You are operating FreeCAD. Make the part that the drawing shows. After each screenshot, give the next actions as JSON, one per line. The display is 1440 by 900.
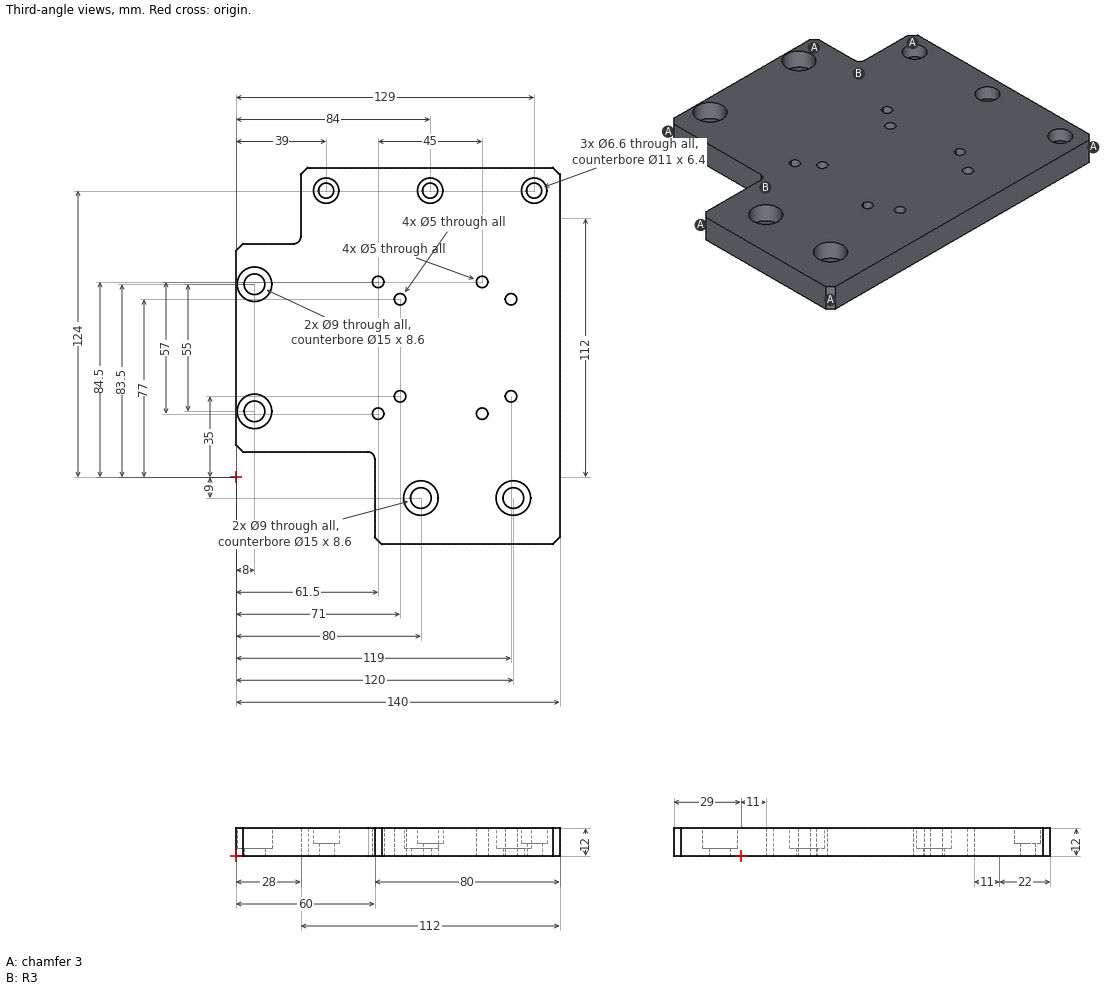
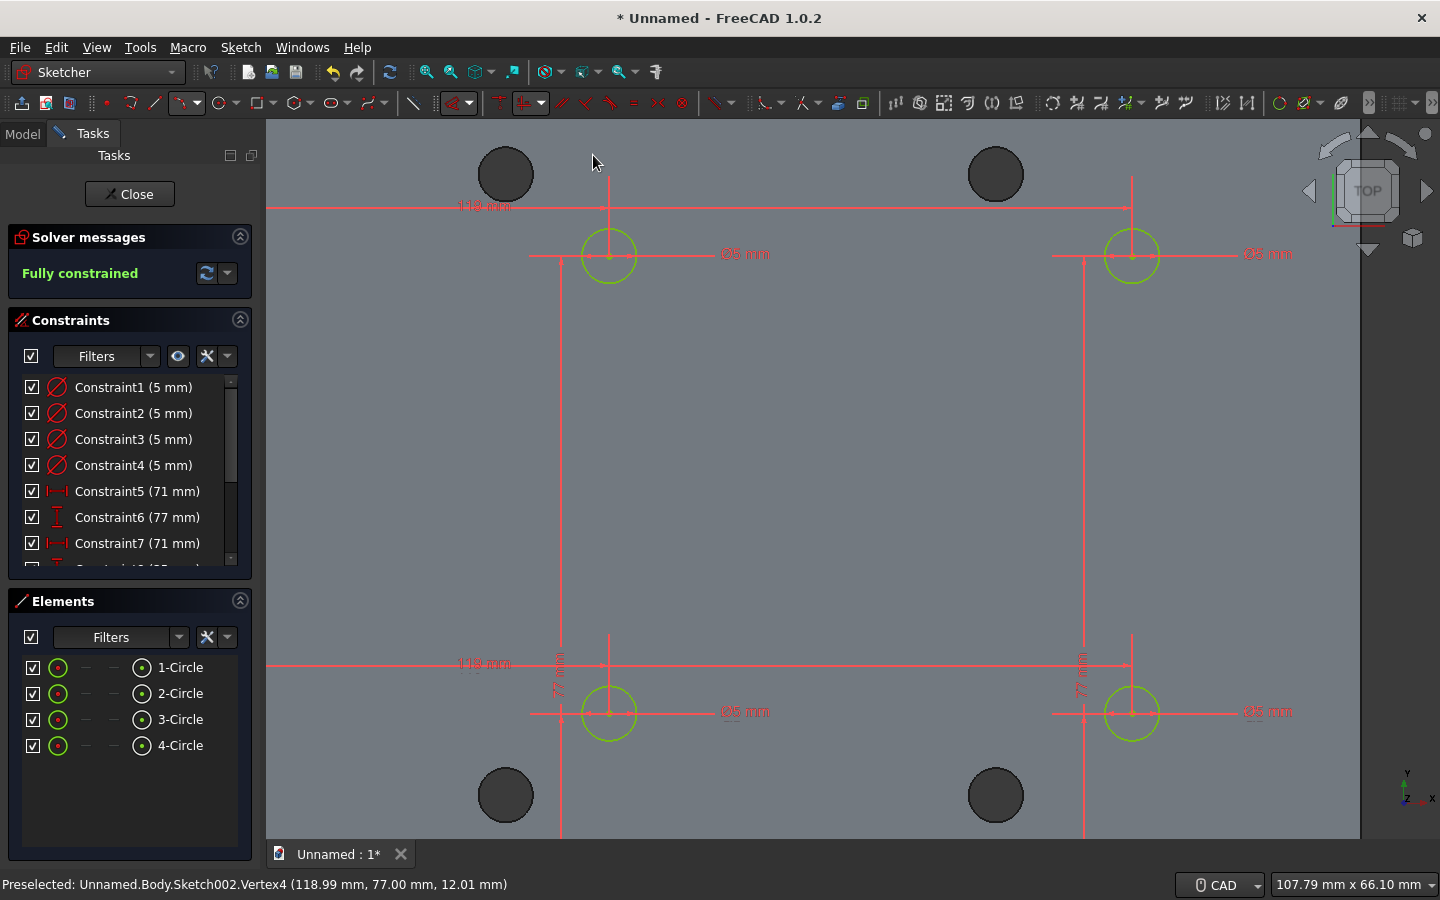
{"action": "left_click", "coordinate": [130, 194]}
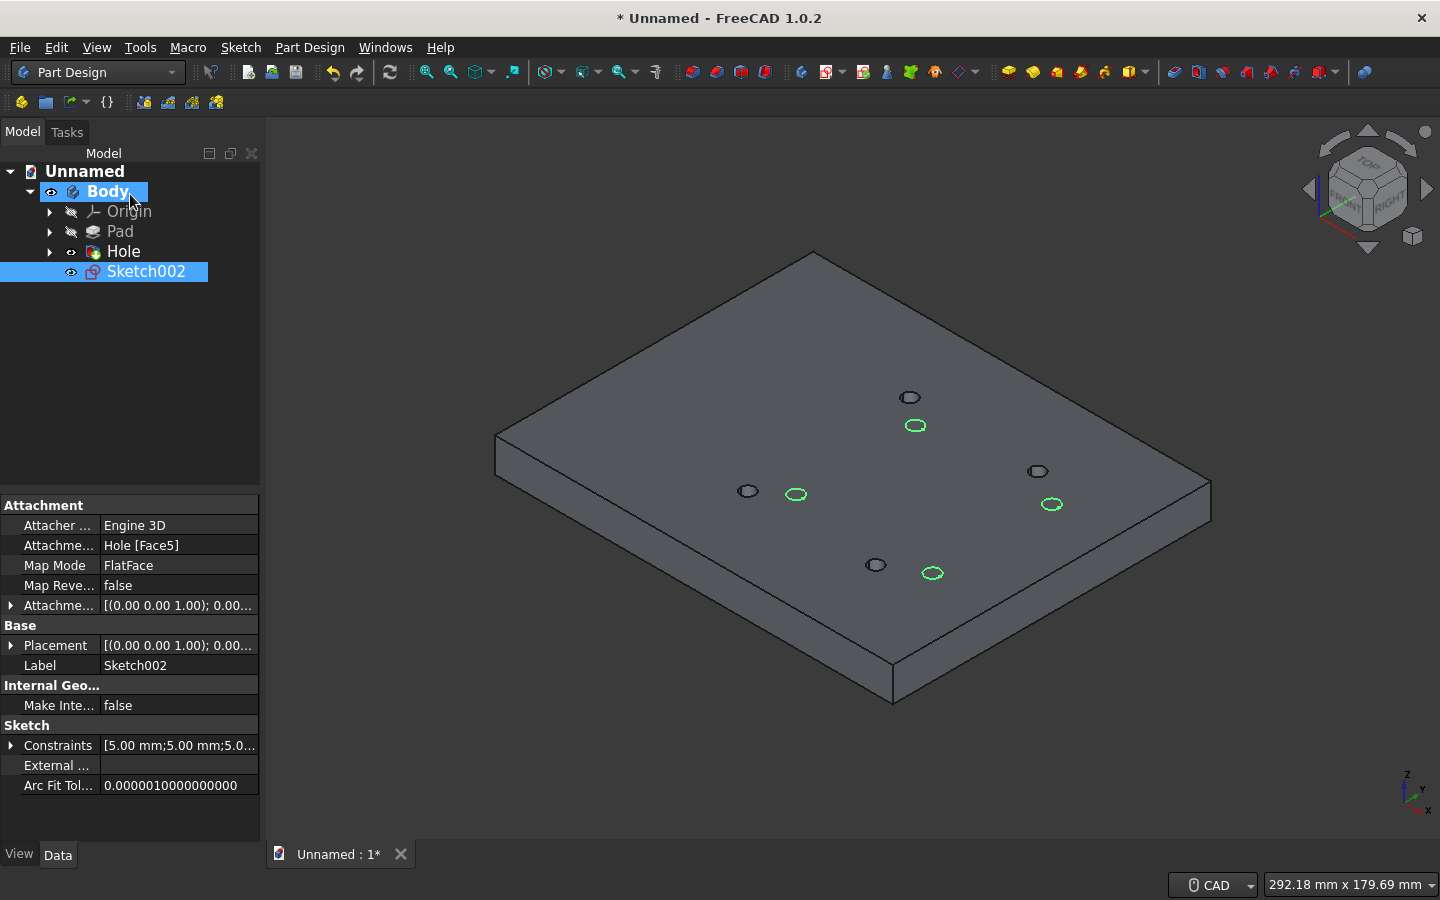
{"action": "left_click", "coordinate": [1200, 72]}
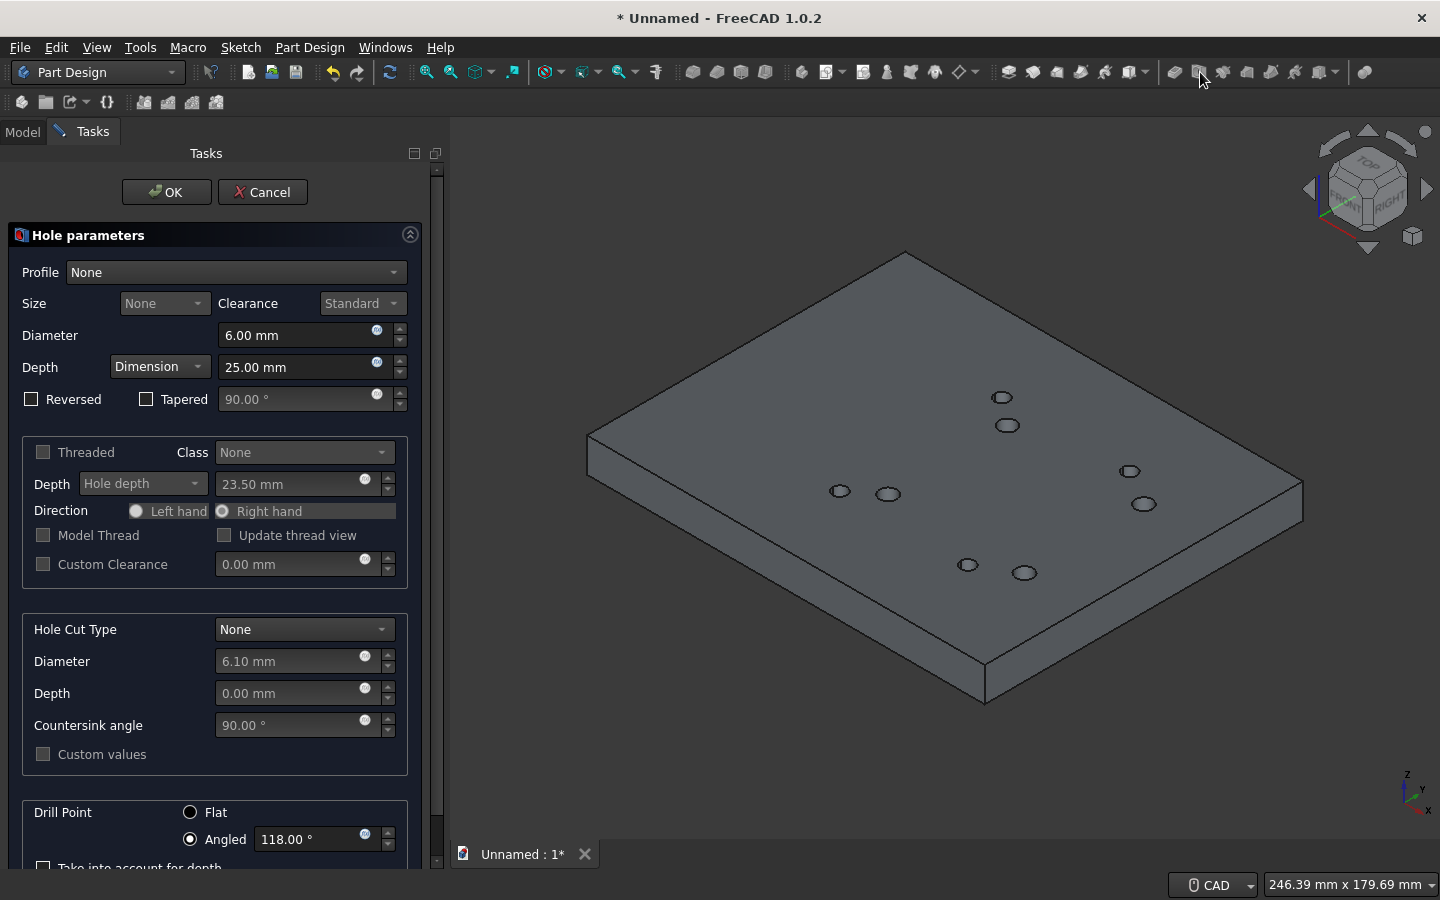
{"action": "triple_click", "coordinate": [305, 335]}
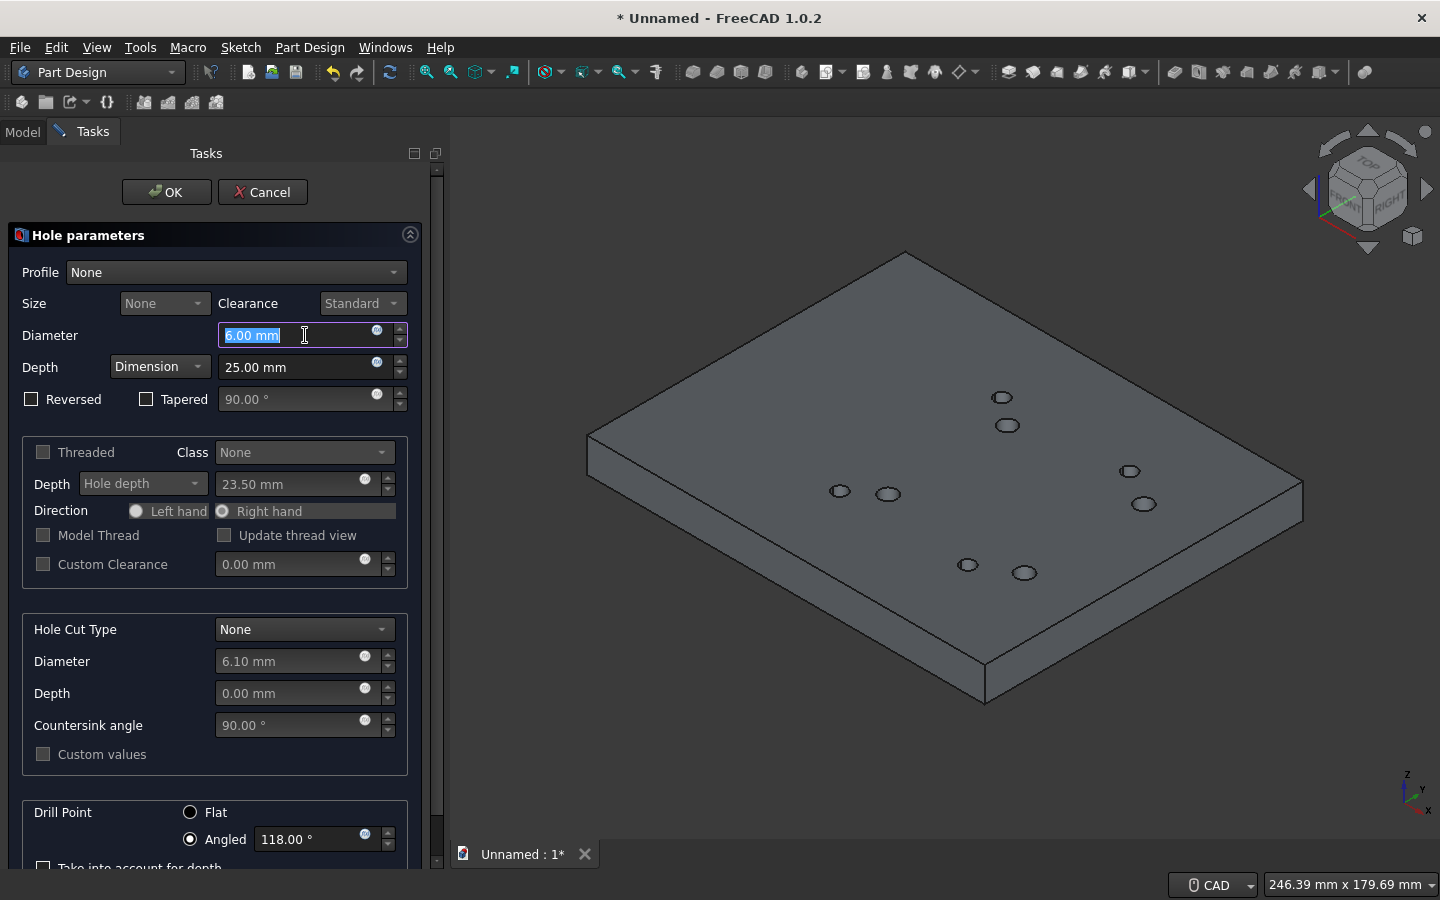
{"action": "type", "text": "5"}
{"action": "key", "text": "Tab"}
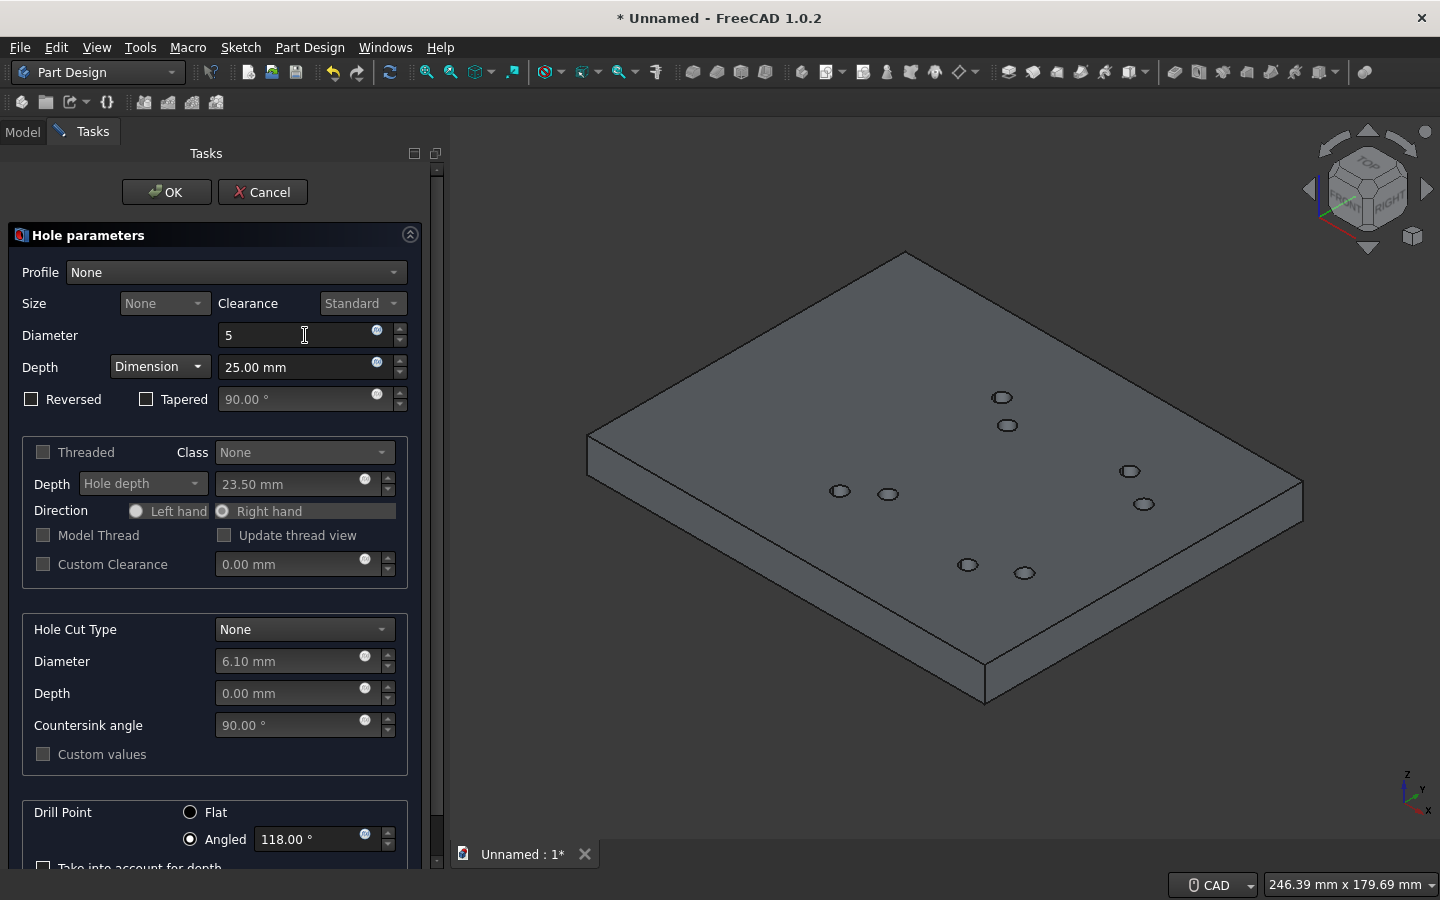
{"action": "left_click", "coordinate": [161, 366]}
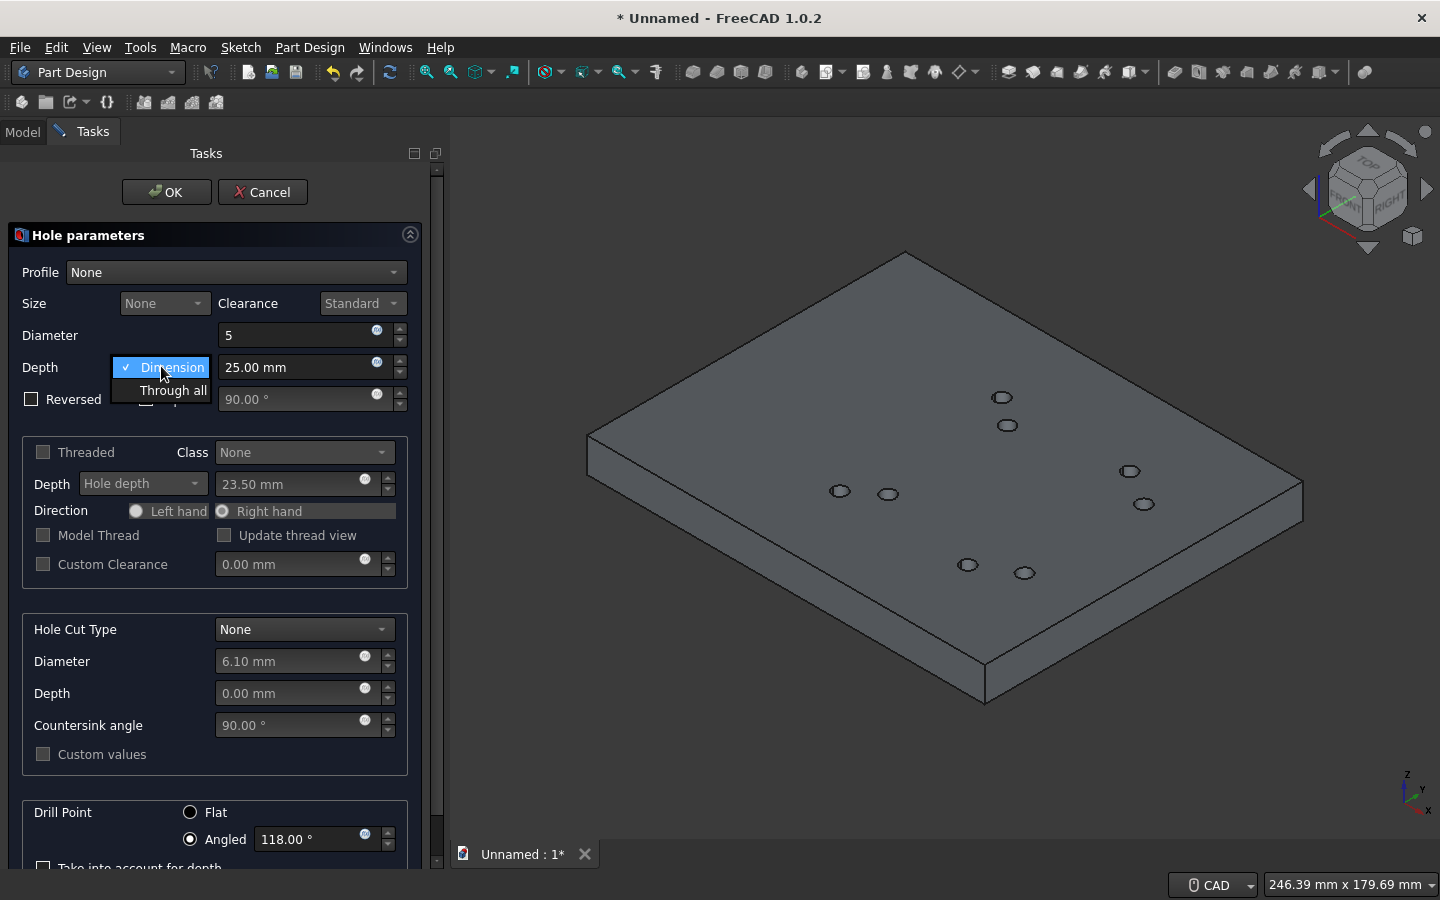
{"action": "left_click", "coordinate": [160, 390]}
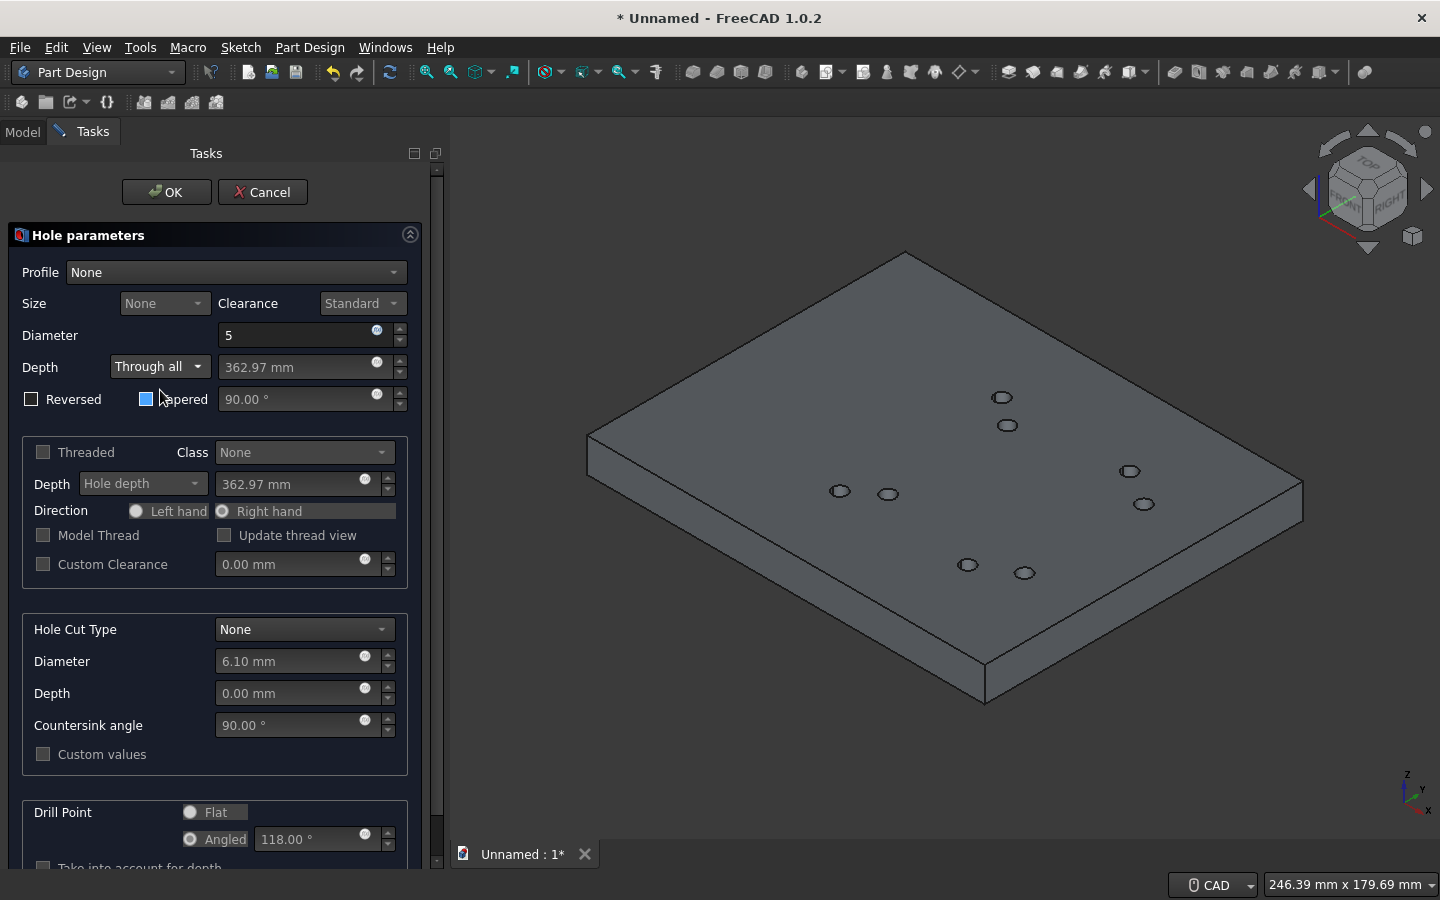
{"action": "left_click", "coordinate": [167, 192]}